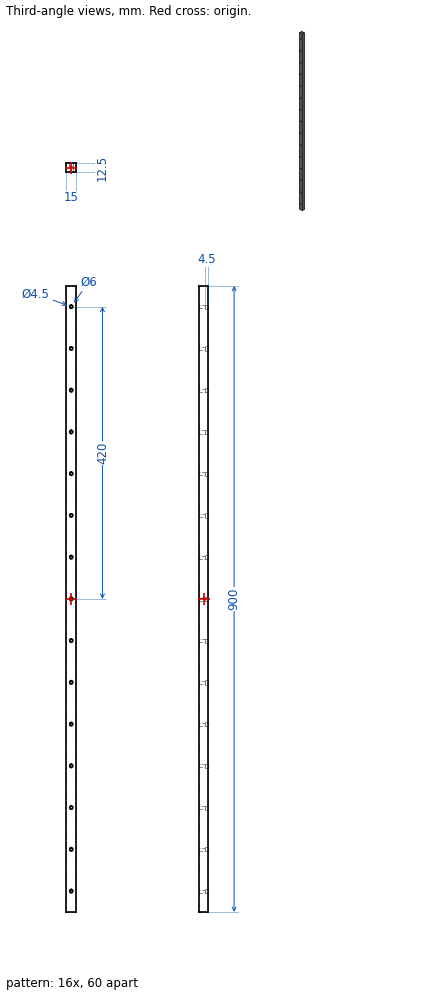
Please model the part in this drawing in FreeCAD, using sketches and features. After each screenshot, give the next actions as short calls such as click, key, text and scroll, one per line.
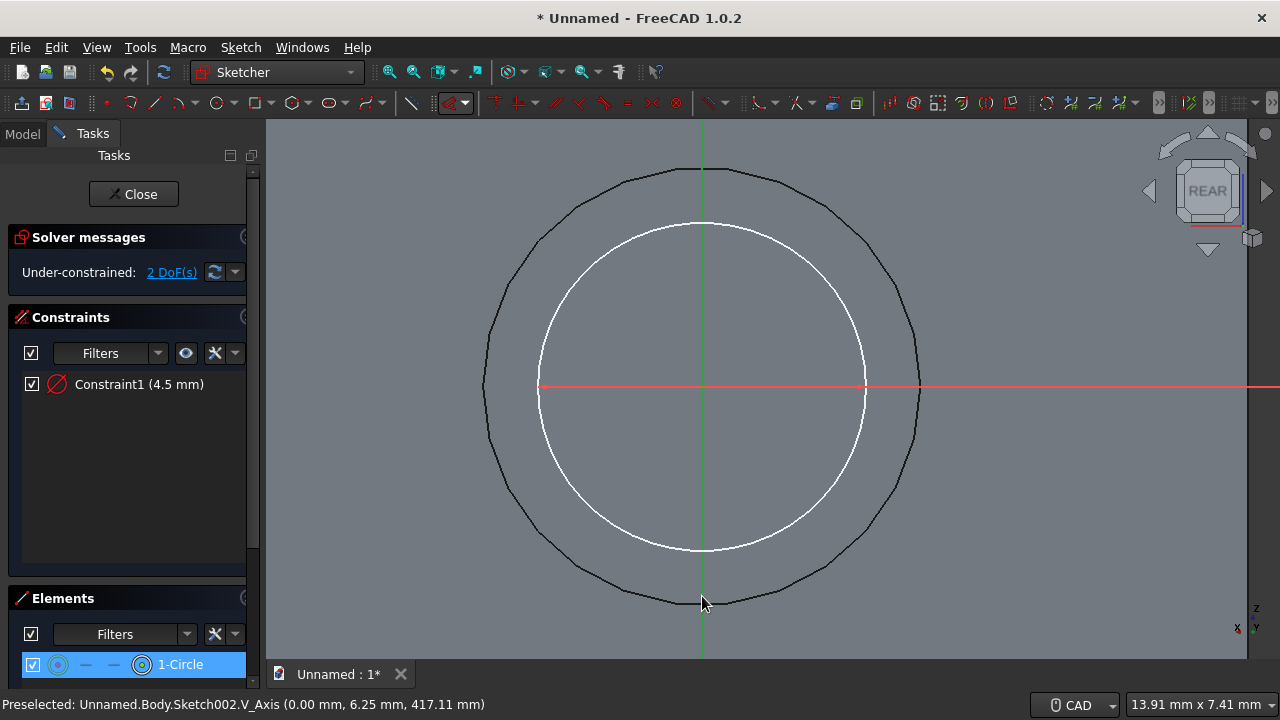
click(496, 104)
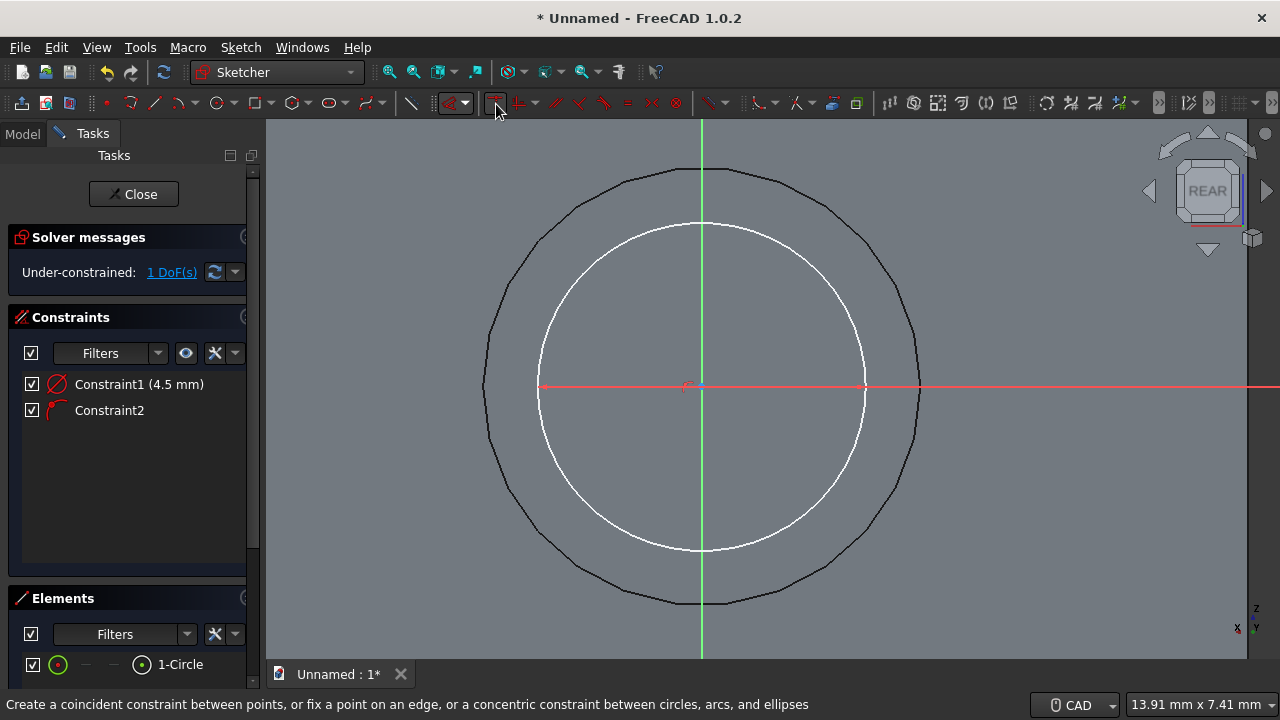
click(702, 387)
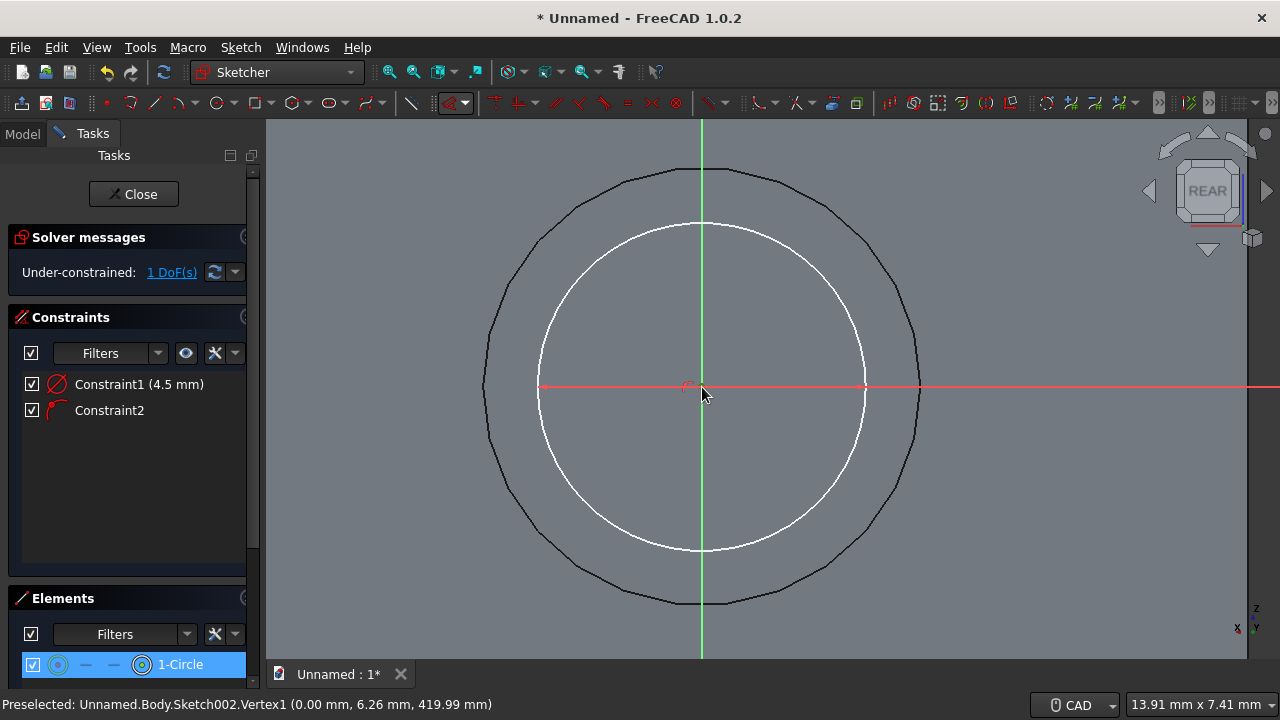
click(468, 104)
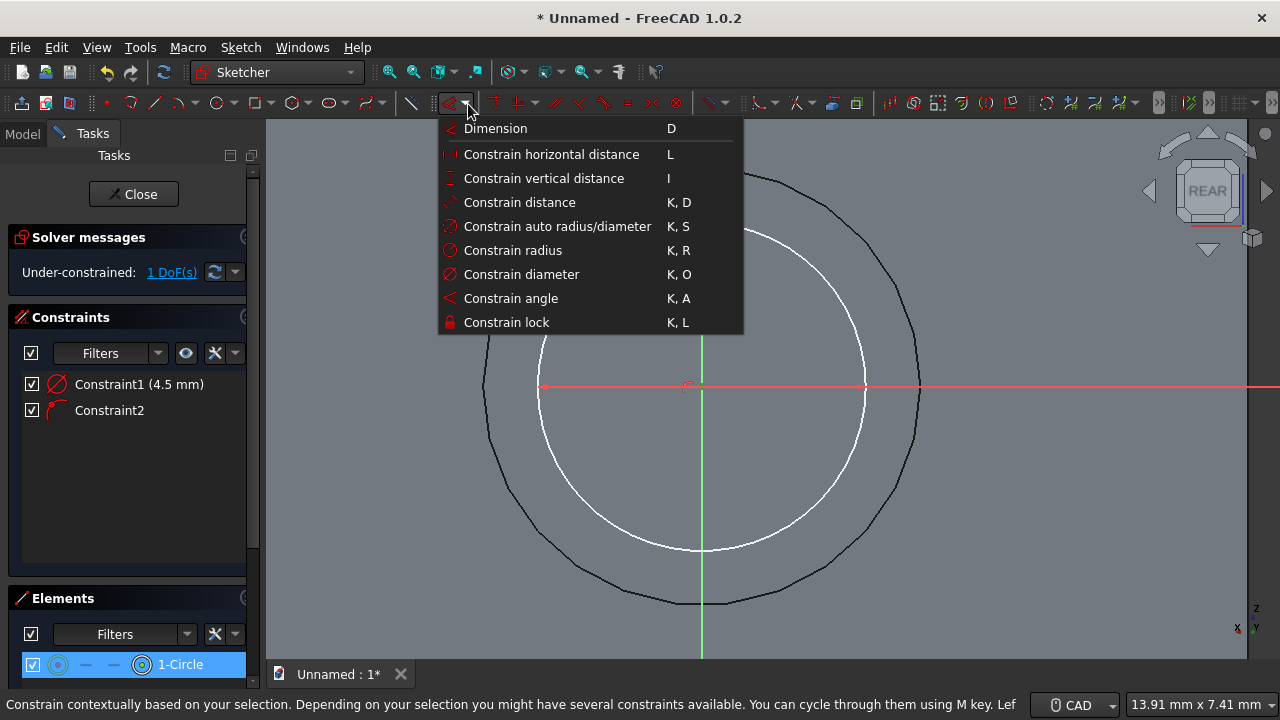
click(591, 178)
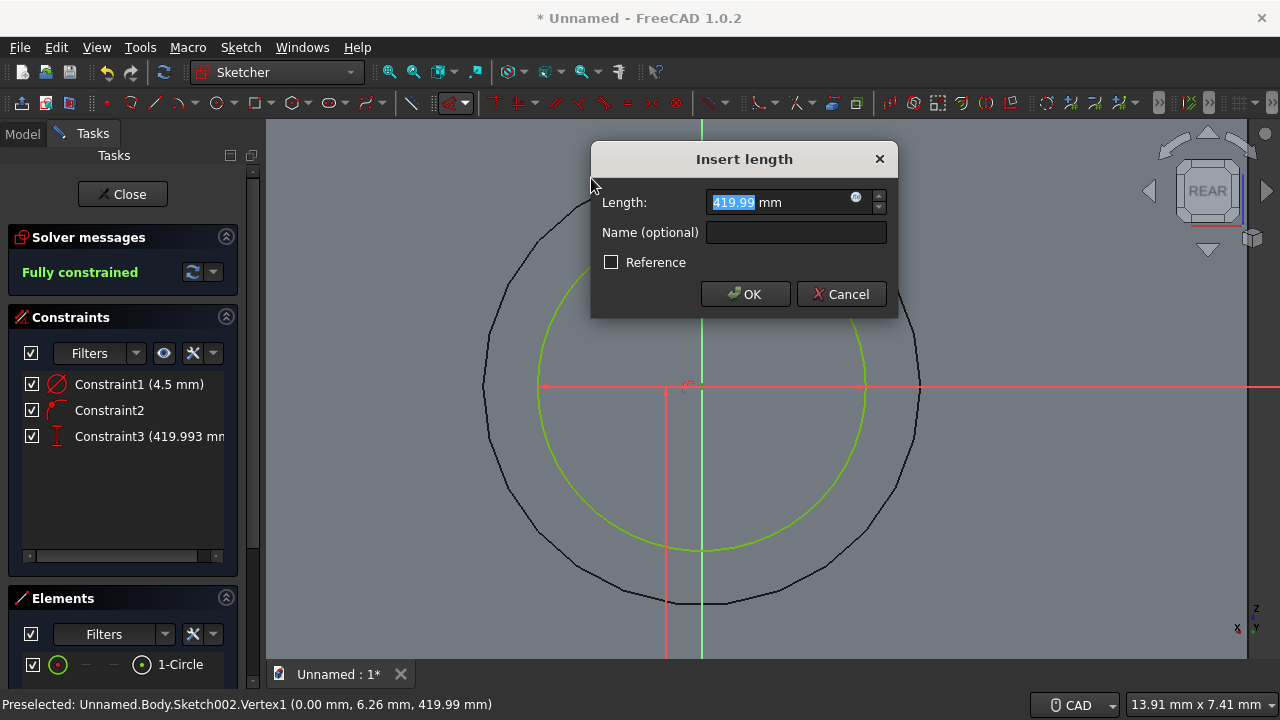
text(420)
key(Return)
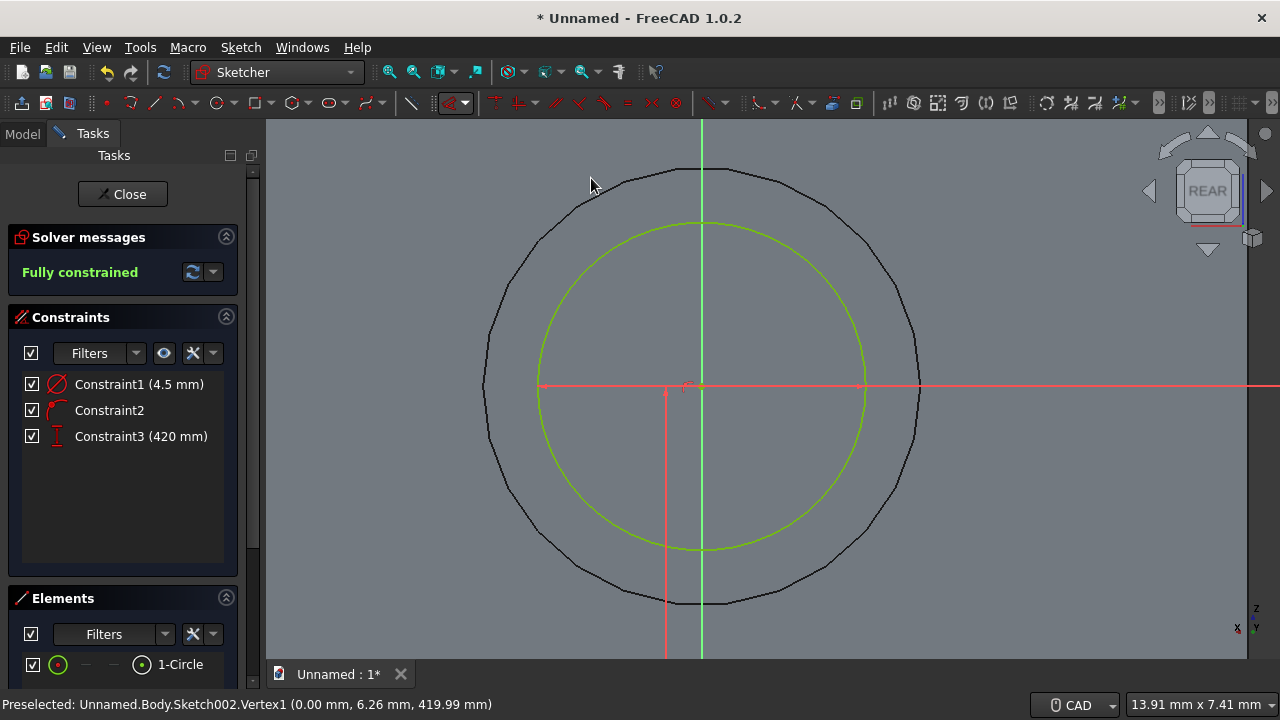
click(123, 194)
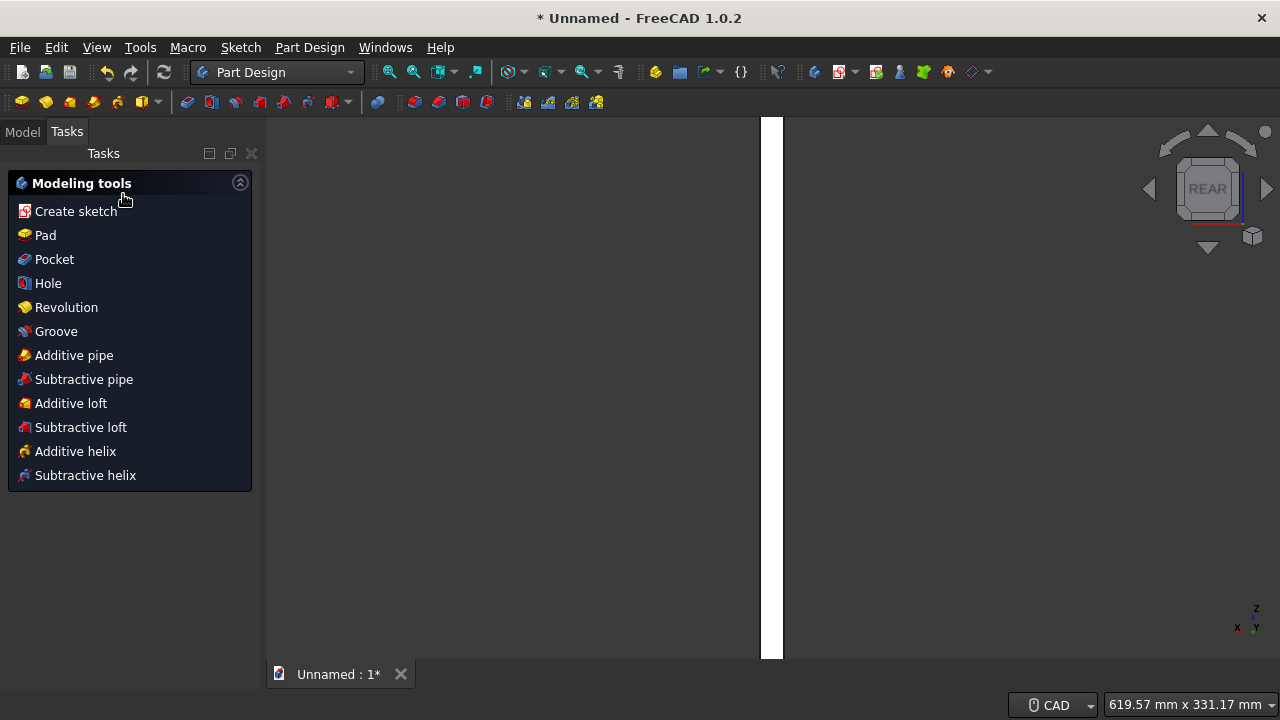
click(188, 102)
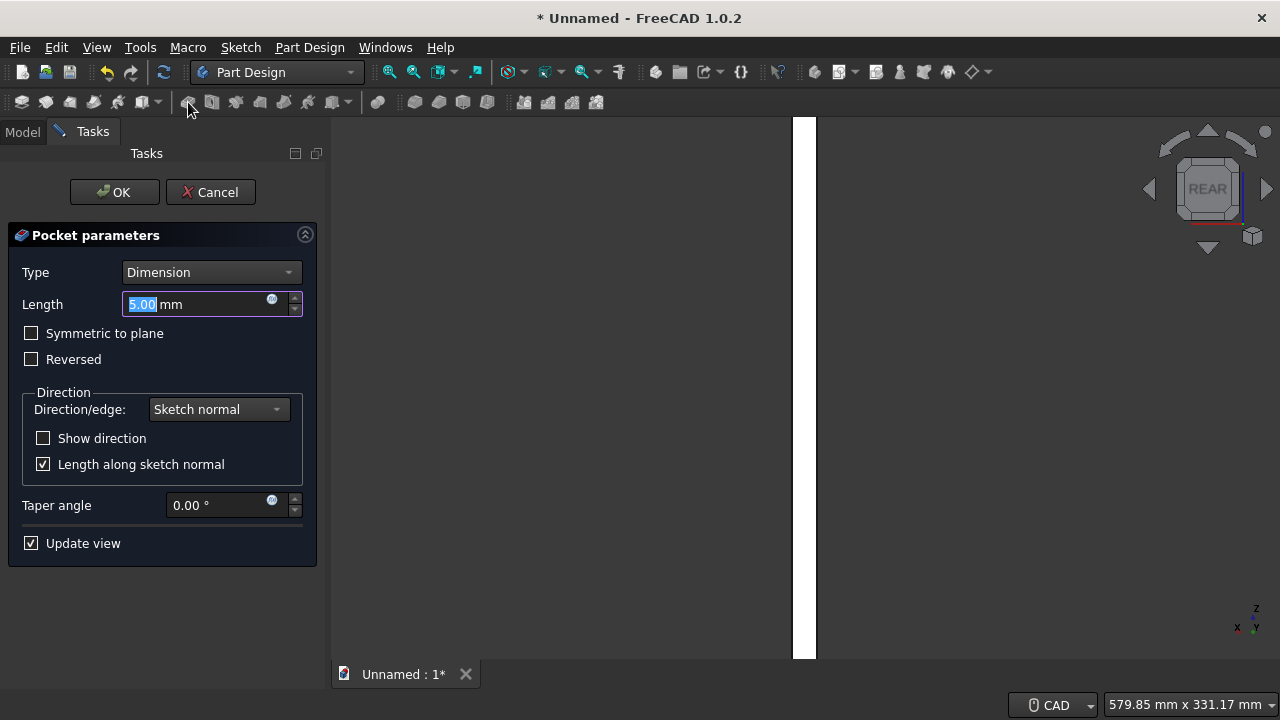
click(212, 272)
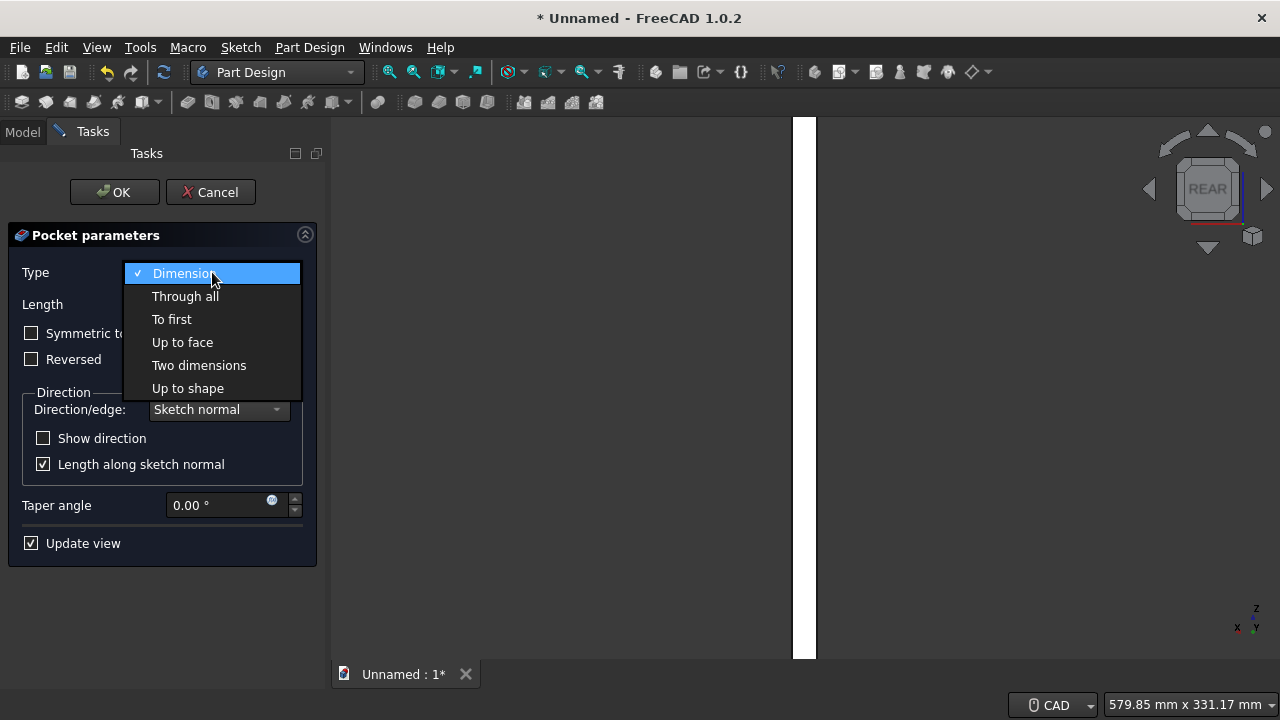
click(212, 296)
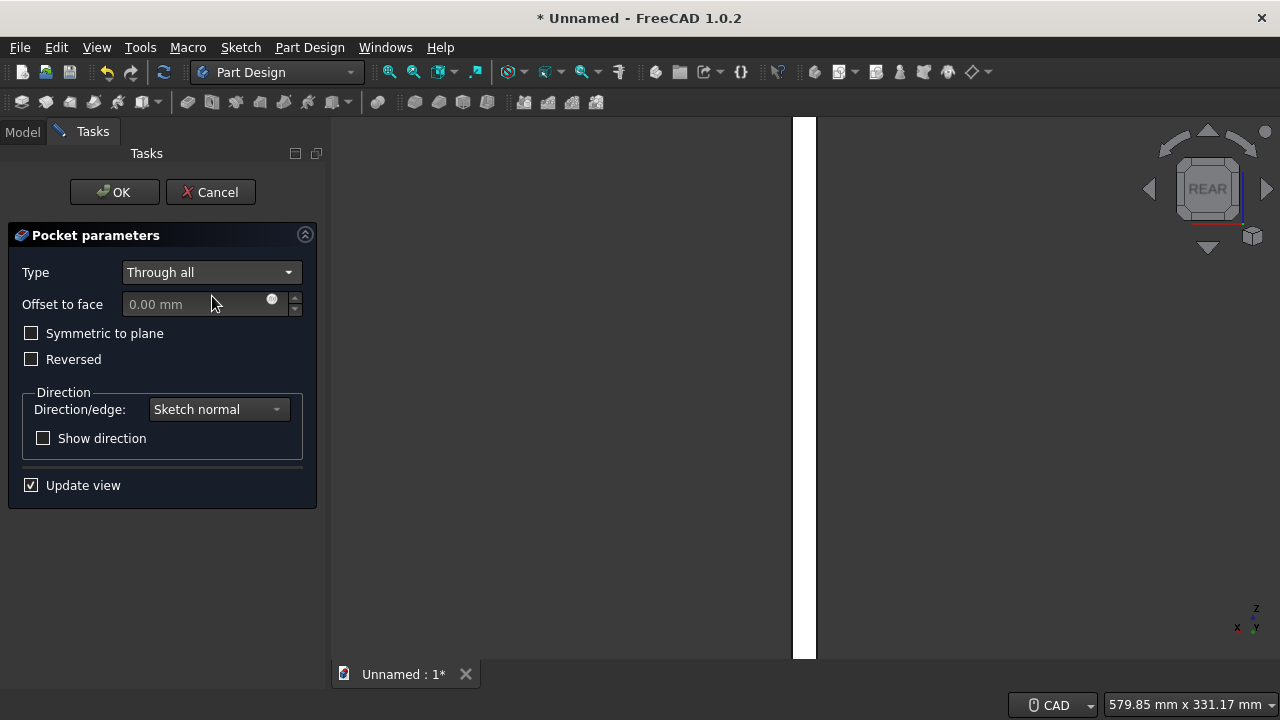
click(115, 192)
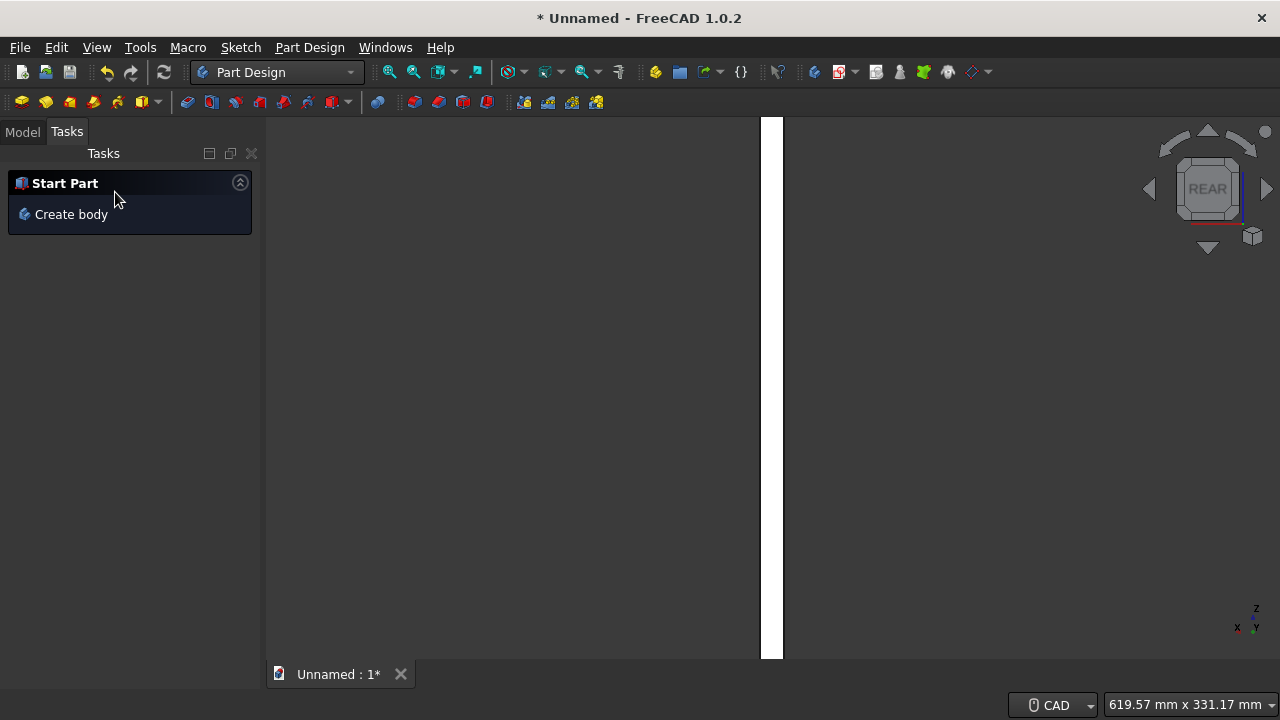
click(390, 72)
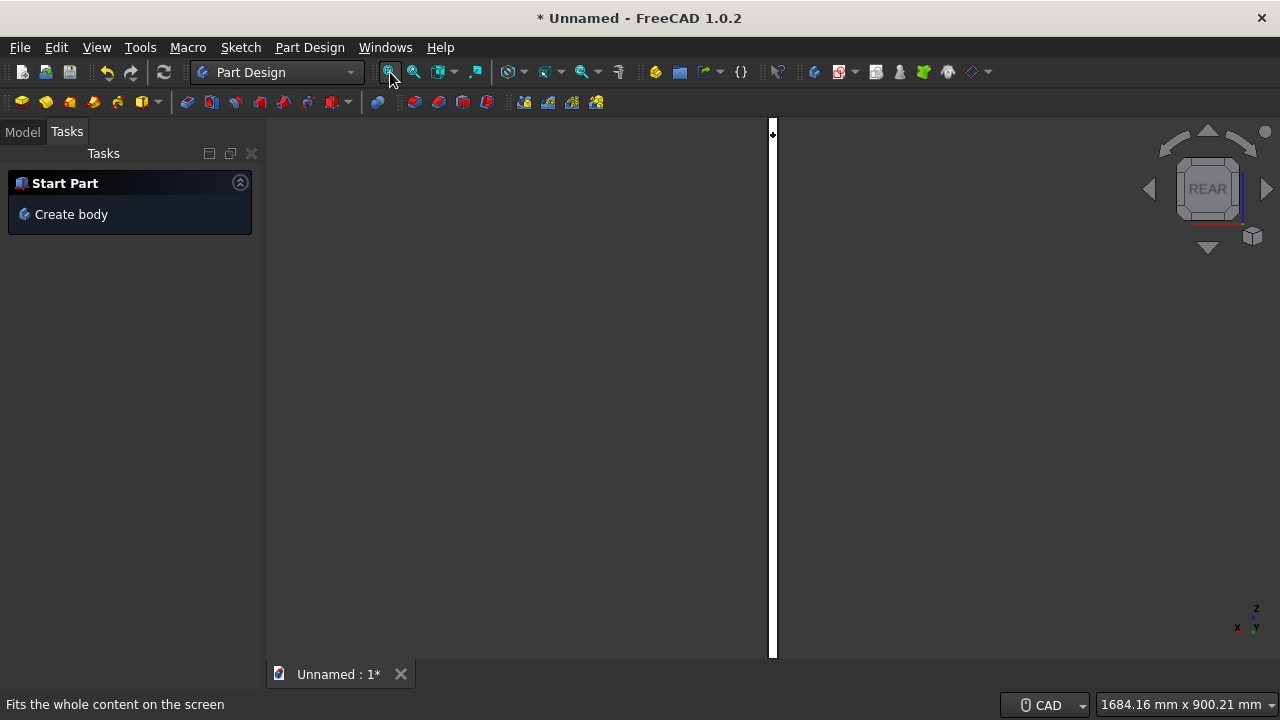
click(23, 131)